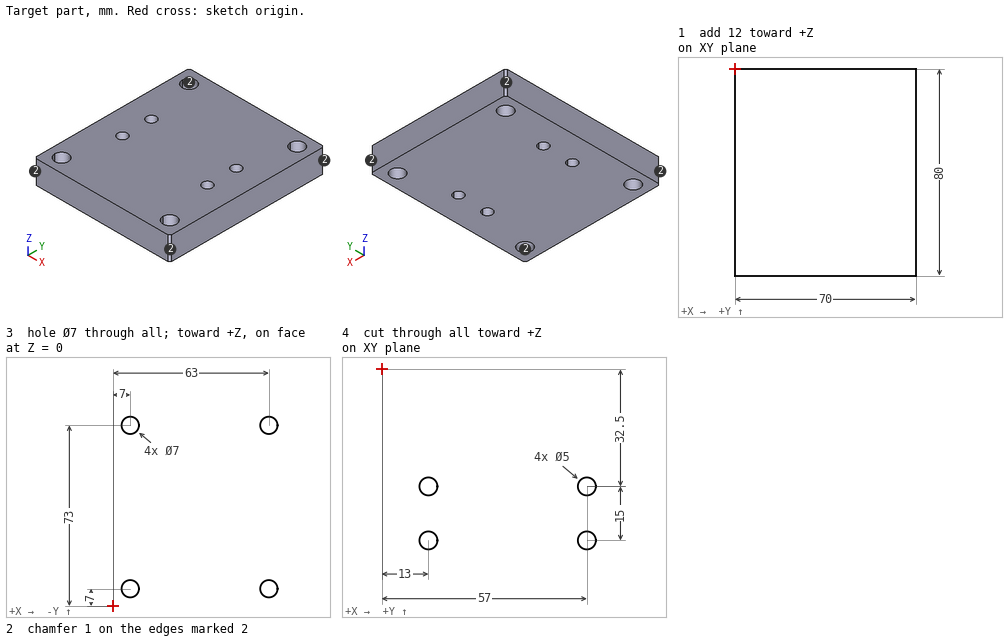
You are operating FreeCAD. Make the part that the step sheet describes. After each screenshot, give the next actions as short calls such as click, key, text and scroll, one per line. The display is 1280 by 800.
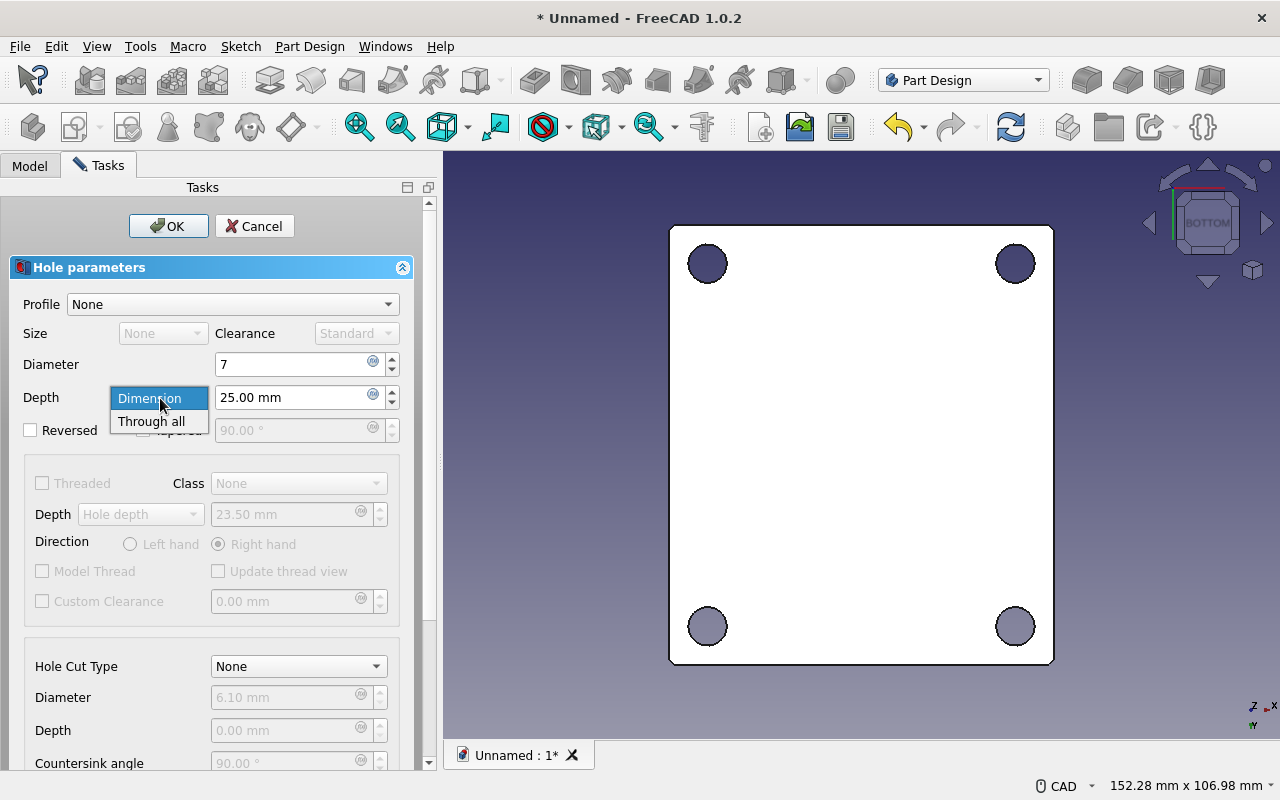
click(158, 422)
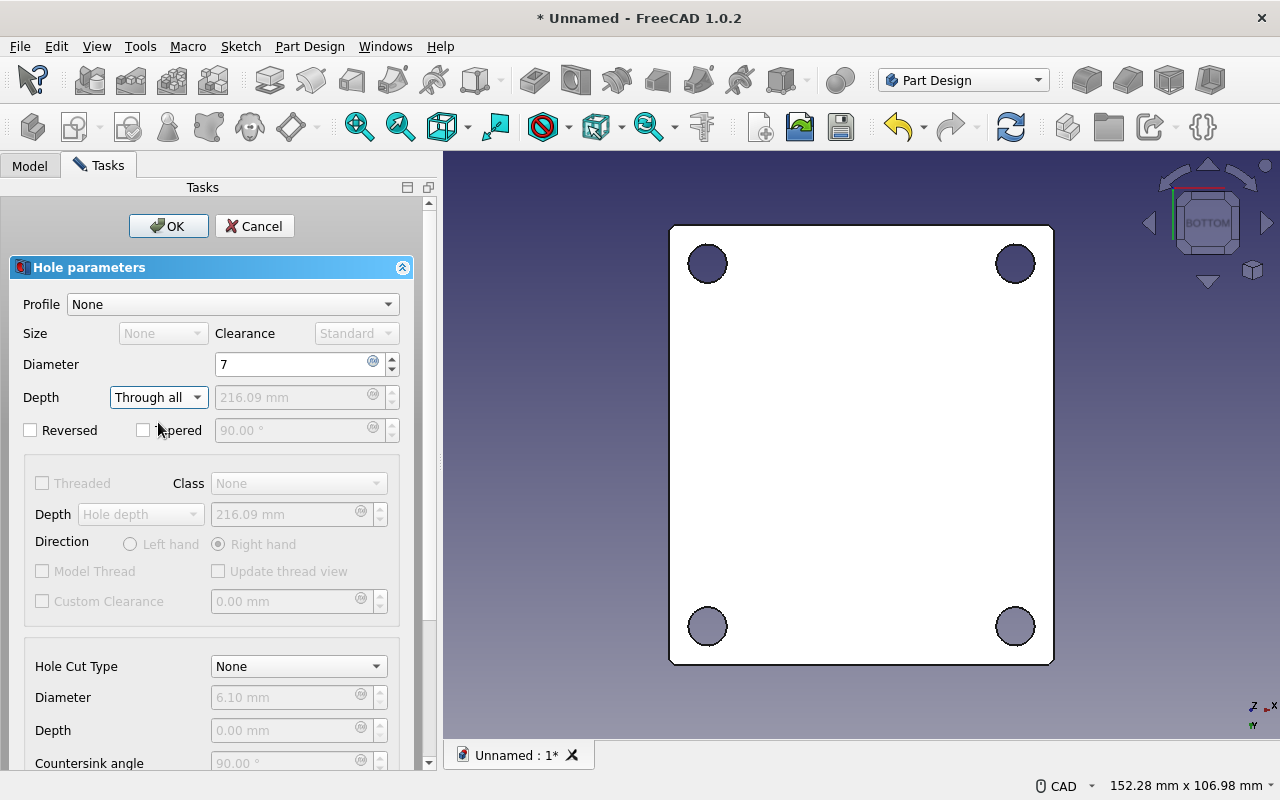
click(169, 226)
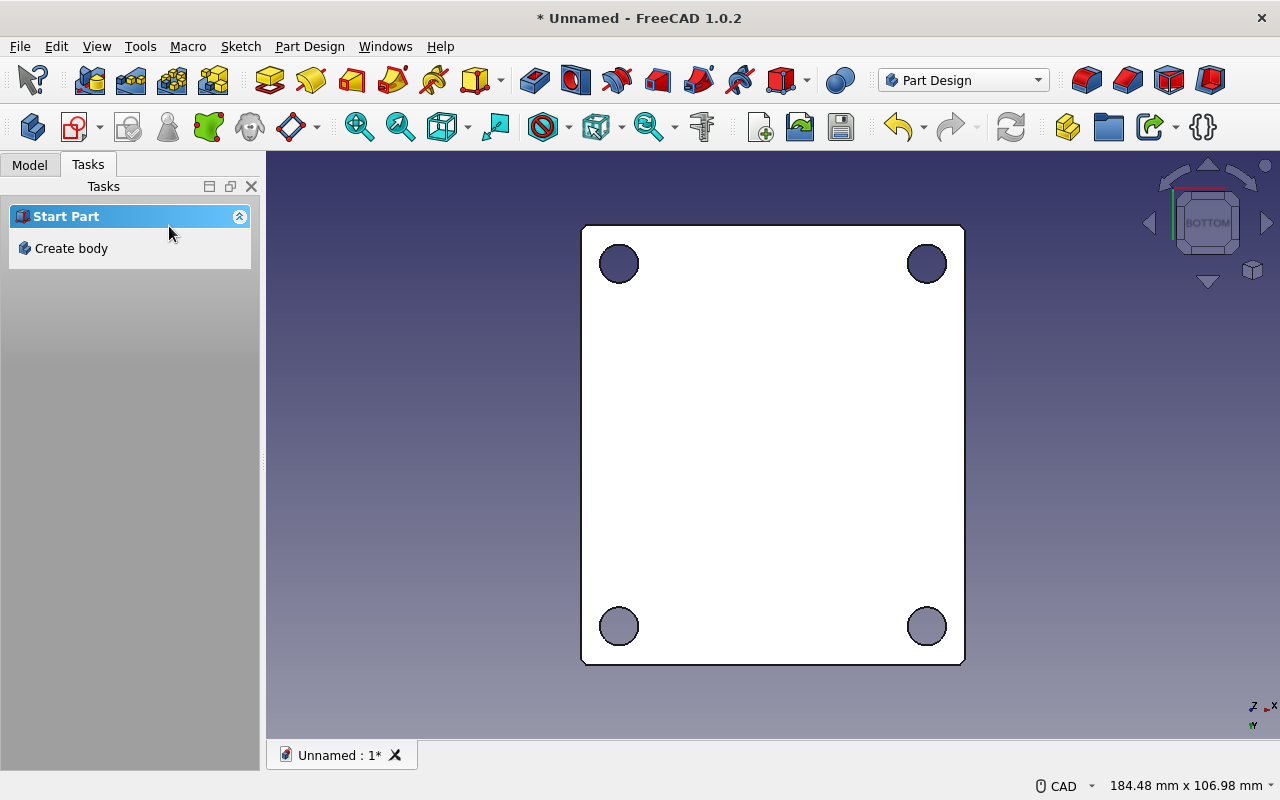
click(74, 128)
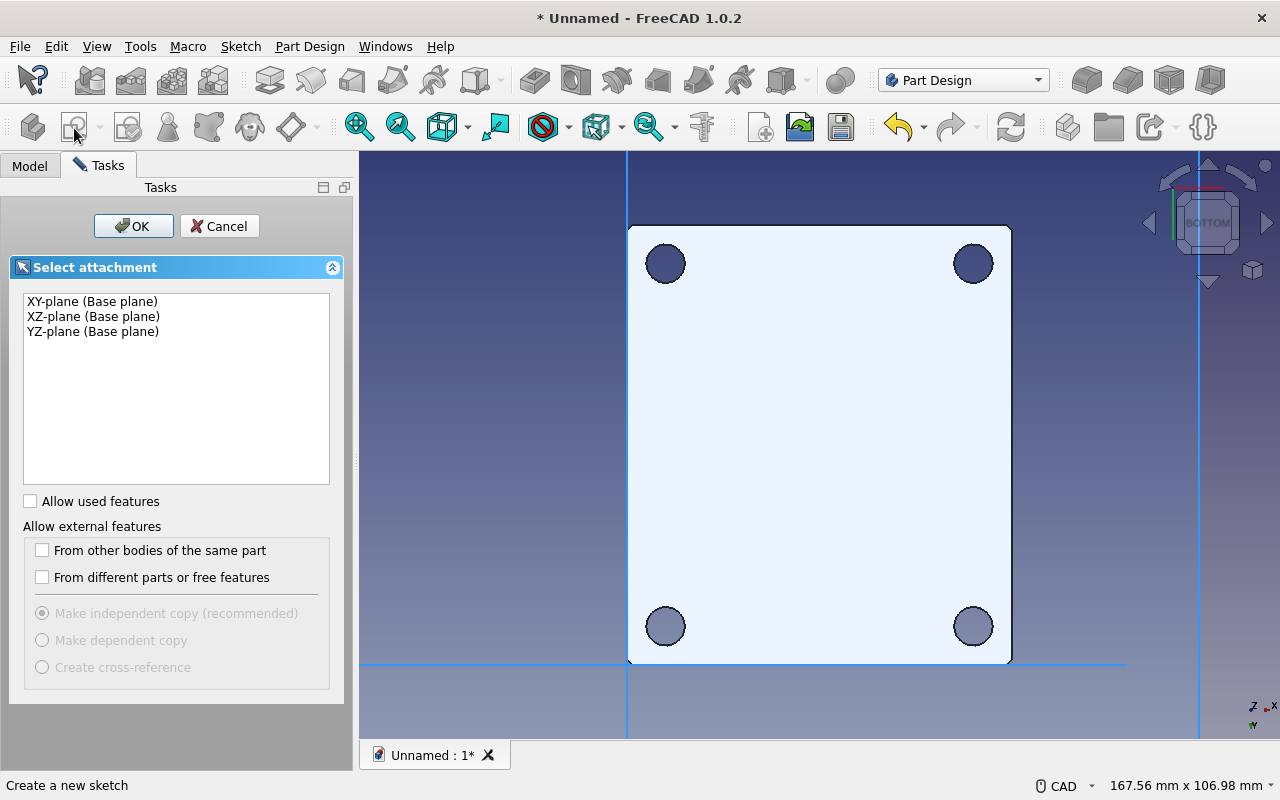
click(84, 302)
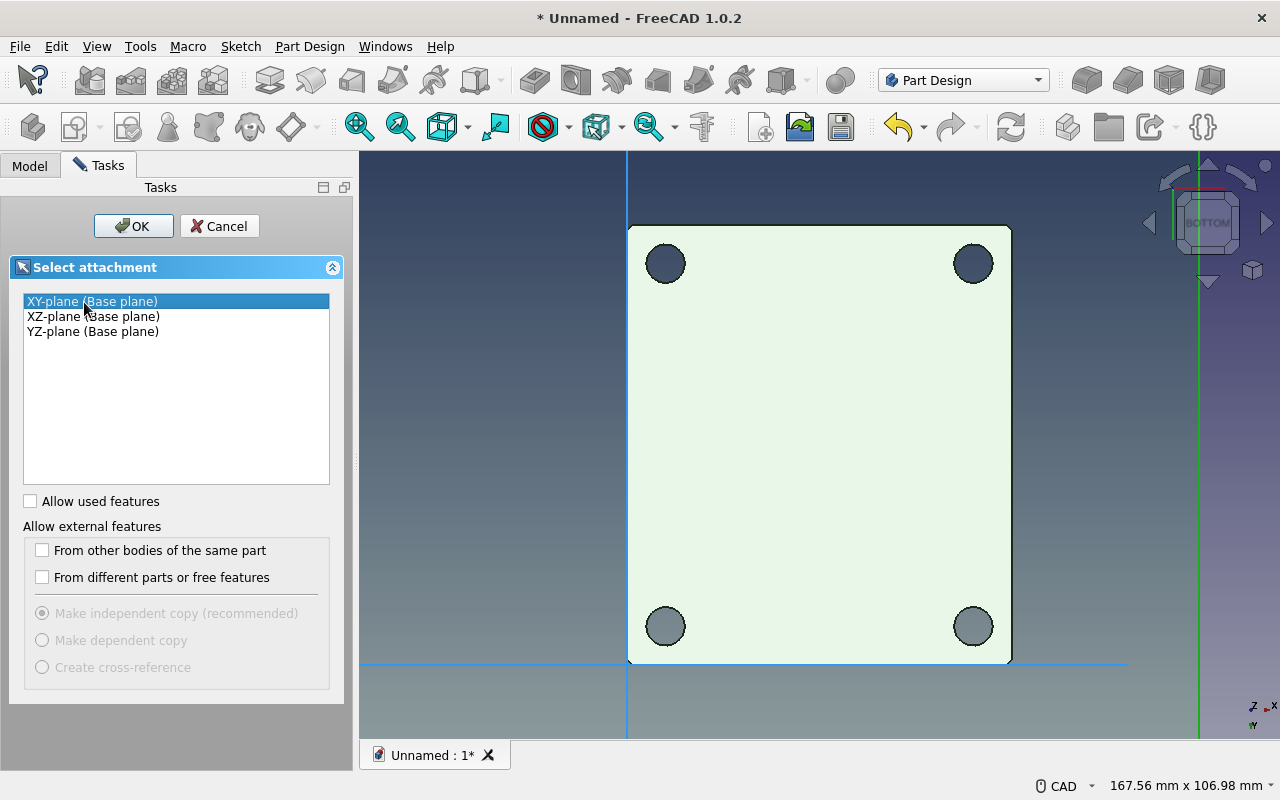
click(134, 226)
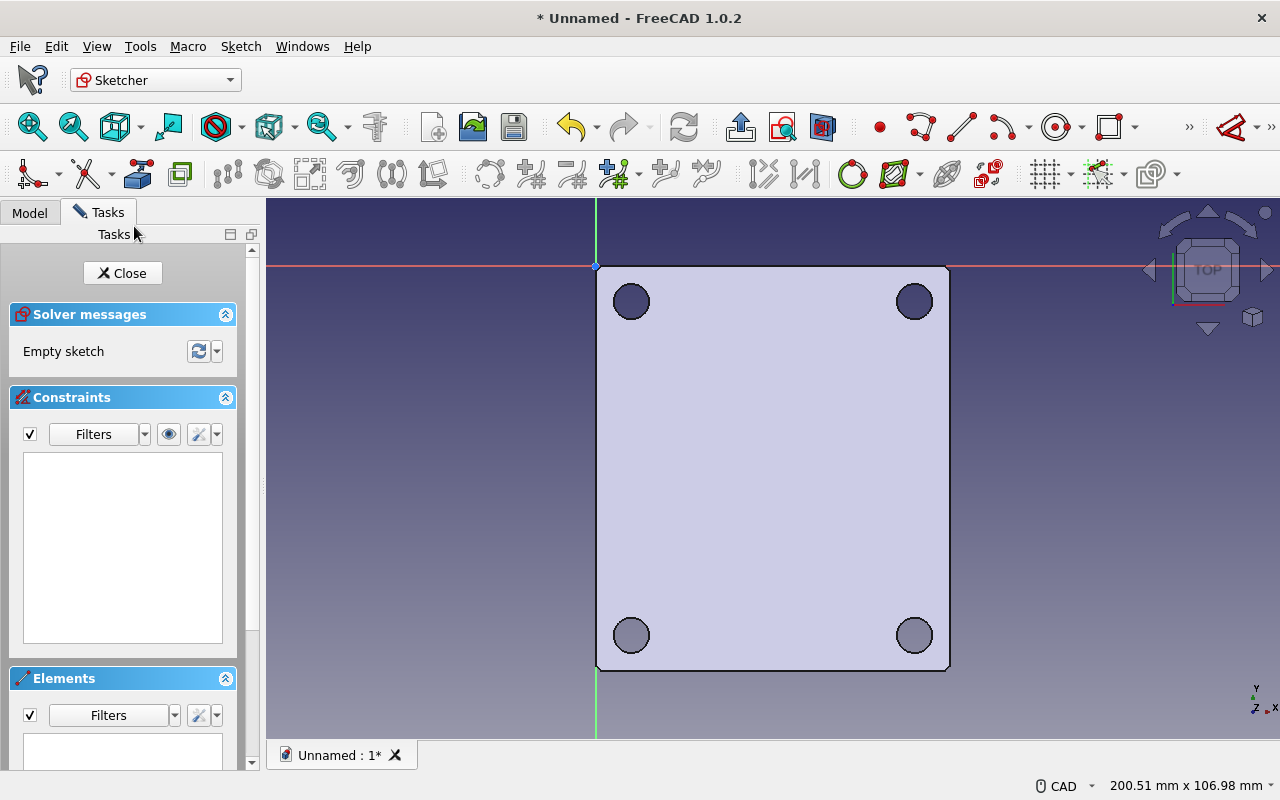
click(823, 128)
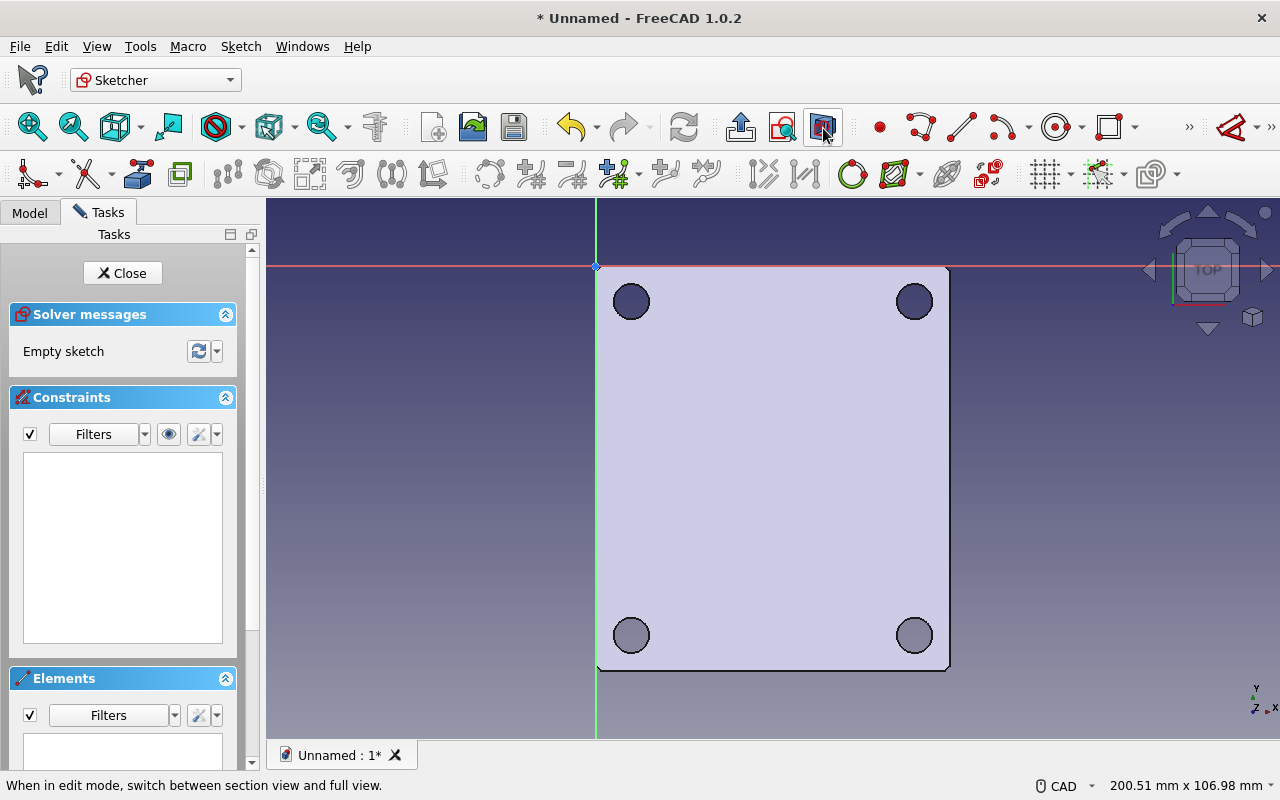
scroll(832, 238, up, 2)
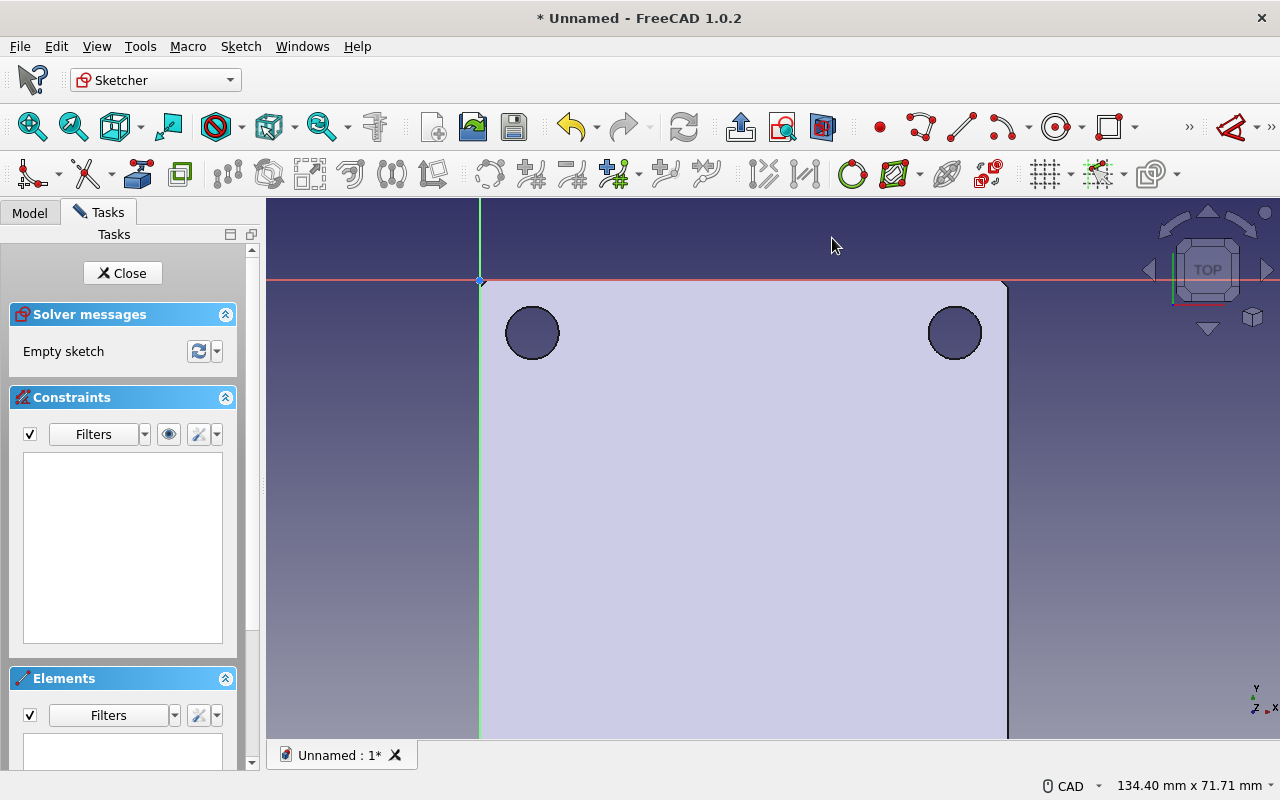
click(1056, 128)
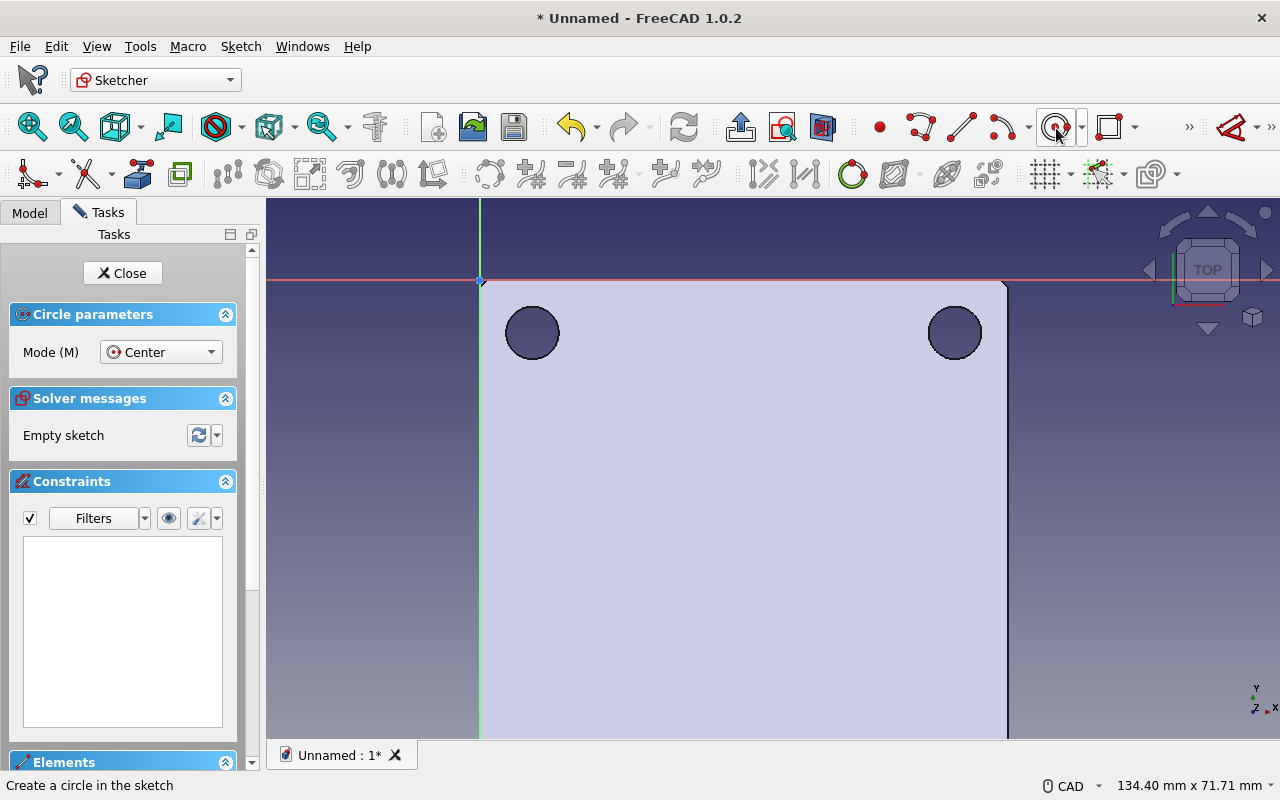
click(910, 525)
move(923, 512)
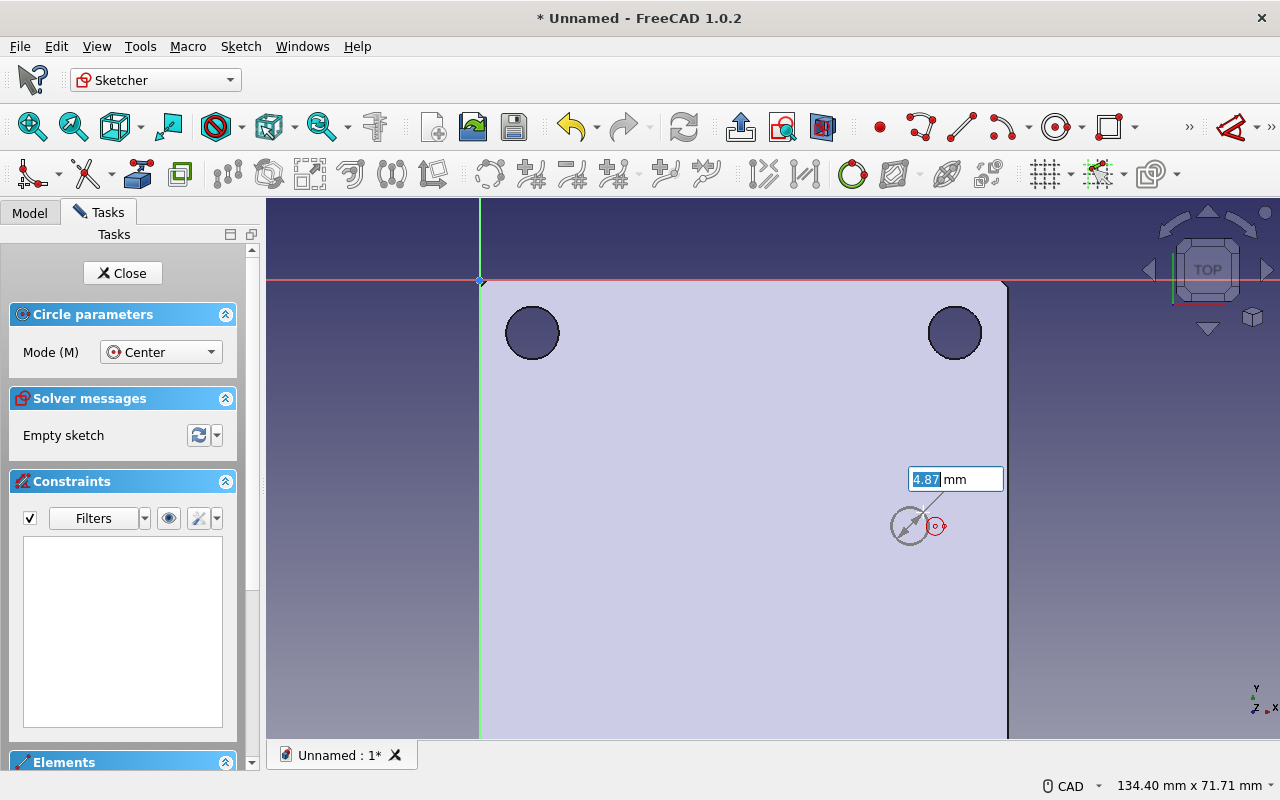
text(5)
key(Return)